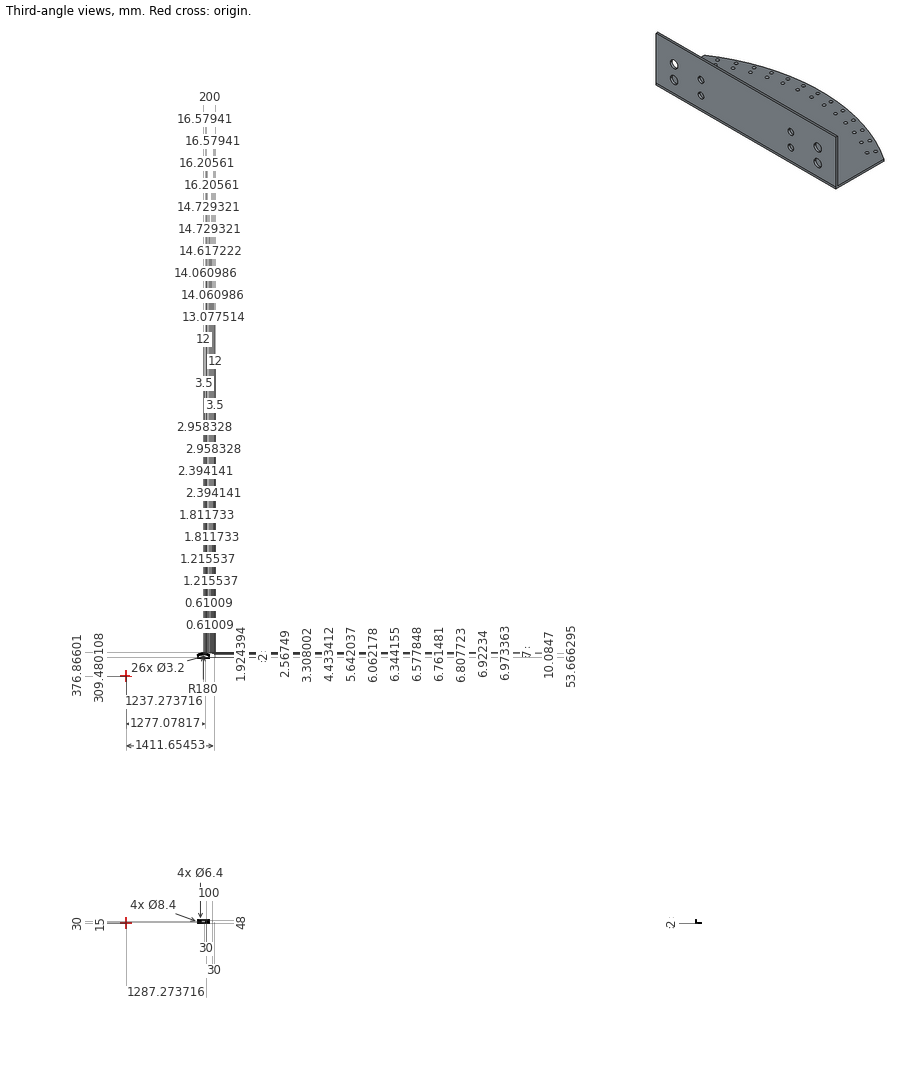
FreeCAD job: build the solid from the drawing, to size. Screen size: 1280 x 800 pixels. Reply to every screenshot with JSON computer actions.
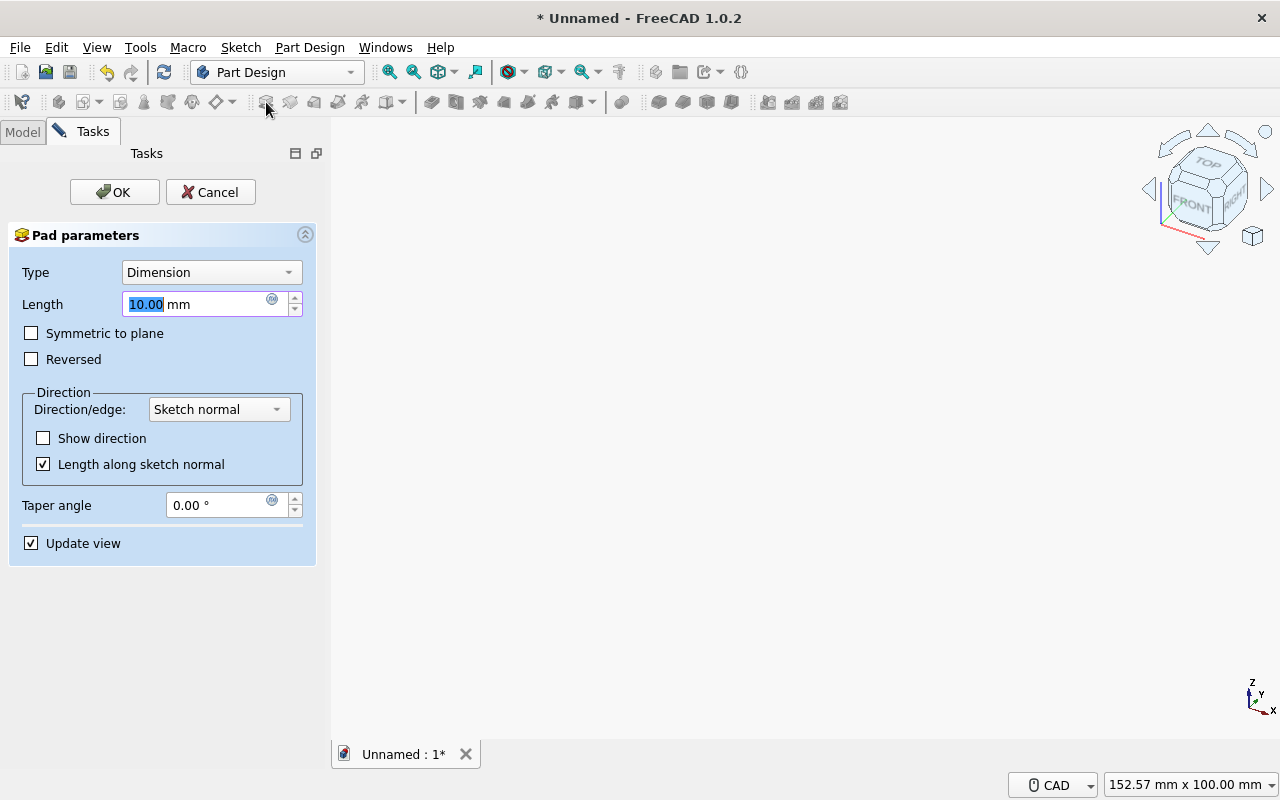
{"action": "type", "text": "2"}
{"action": "key", "text": "Tab"}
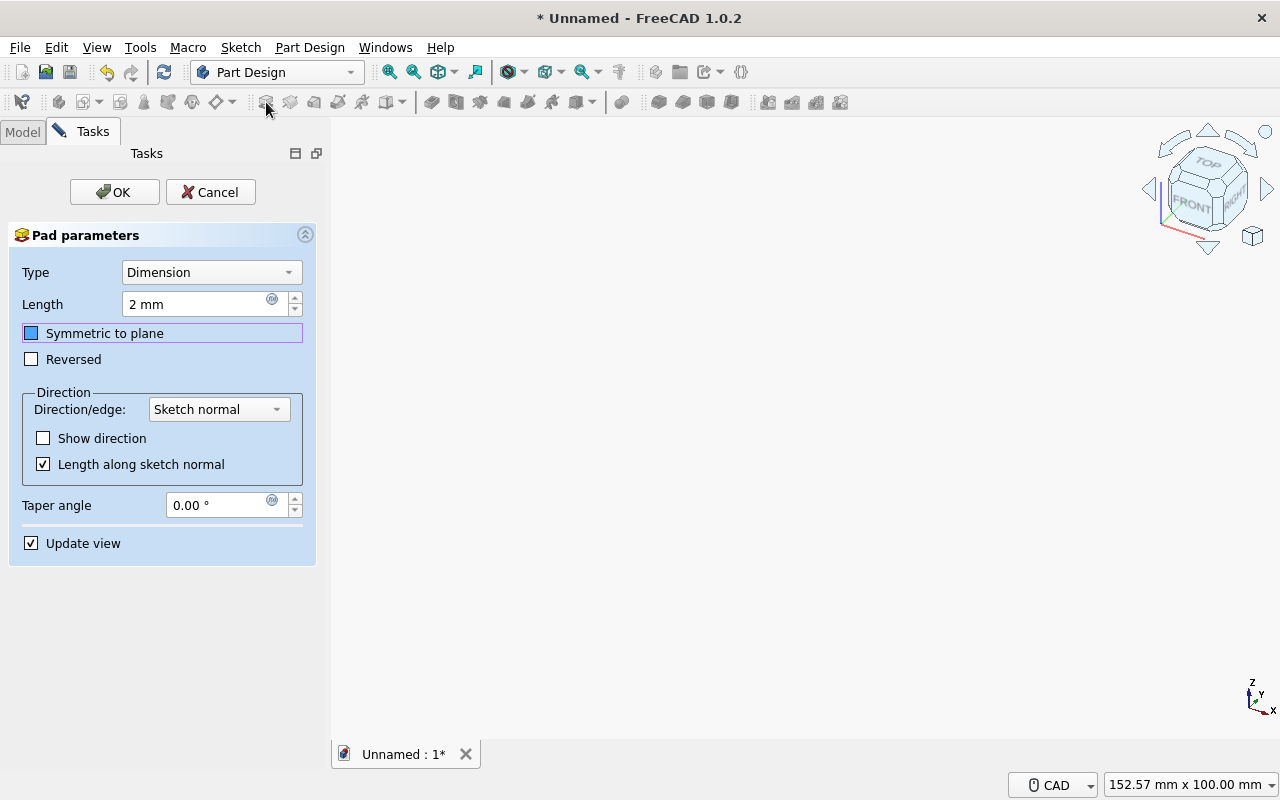
{"action": "left_click", "coordinate": [115, 192]}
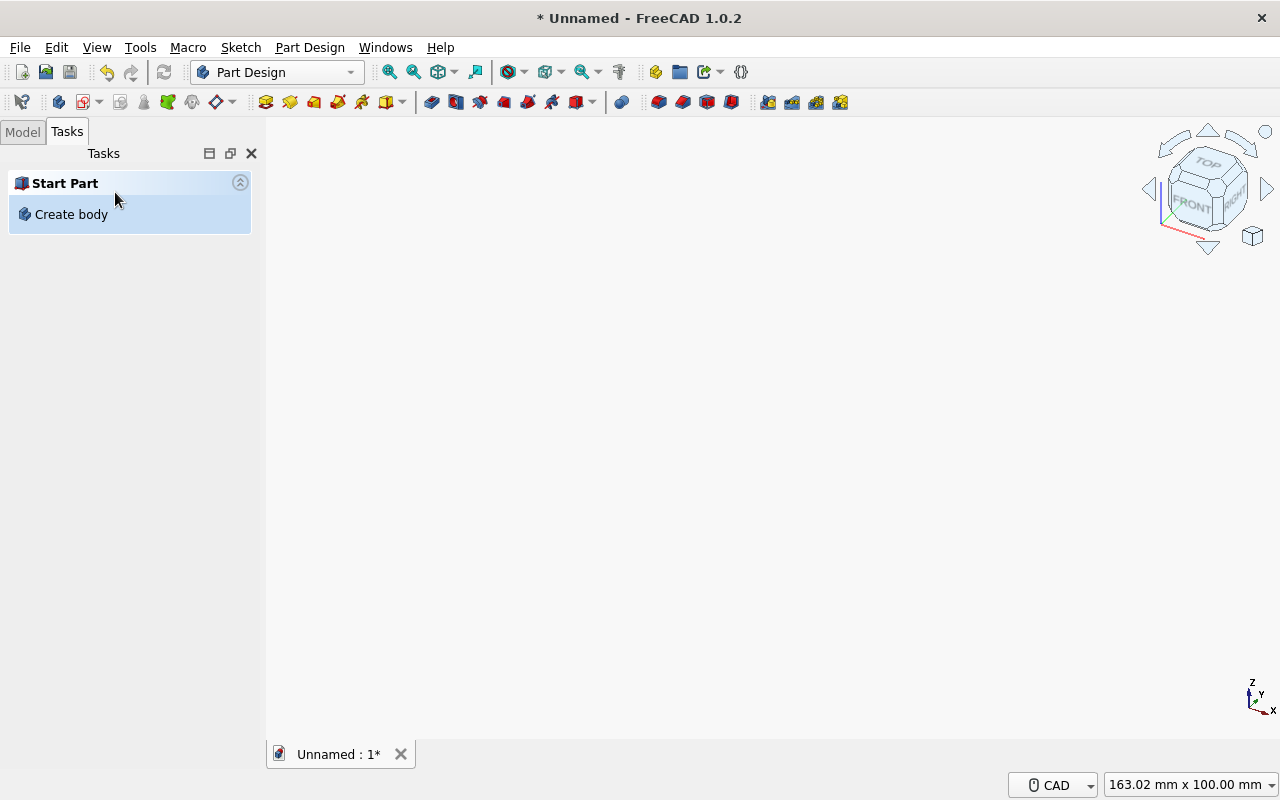
{"action": "key", "text": "v f"}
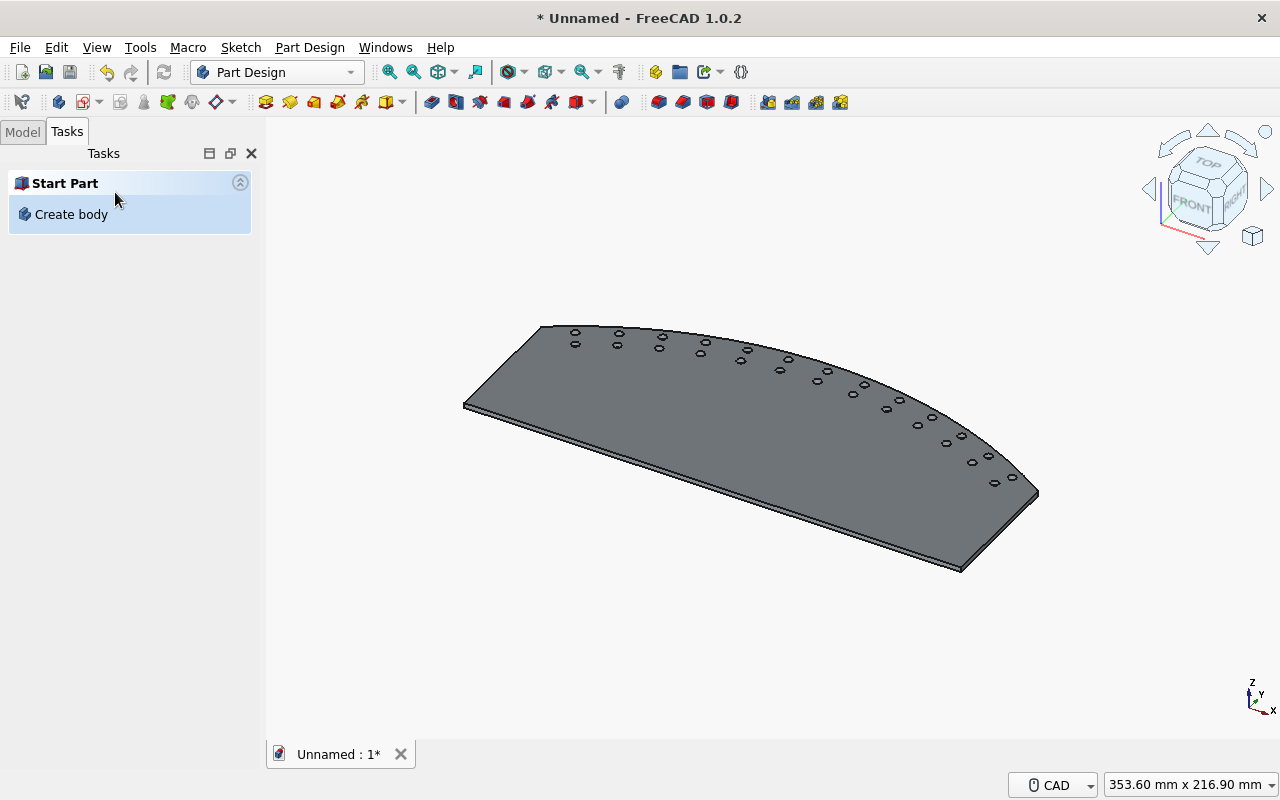
{"action": "left_click", "coordinate": [827, 465]}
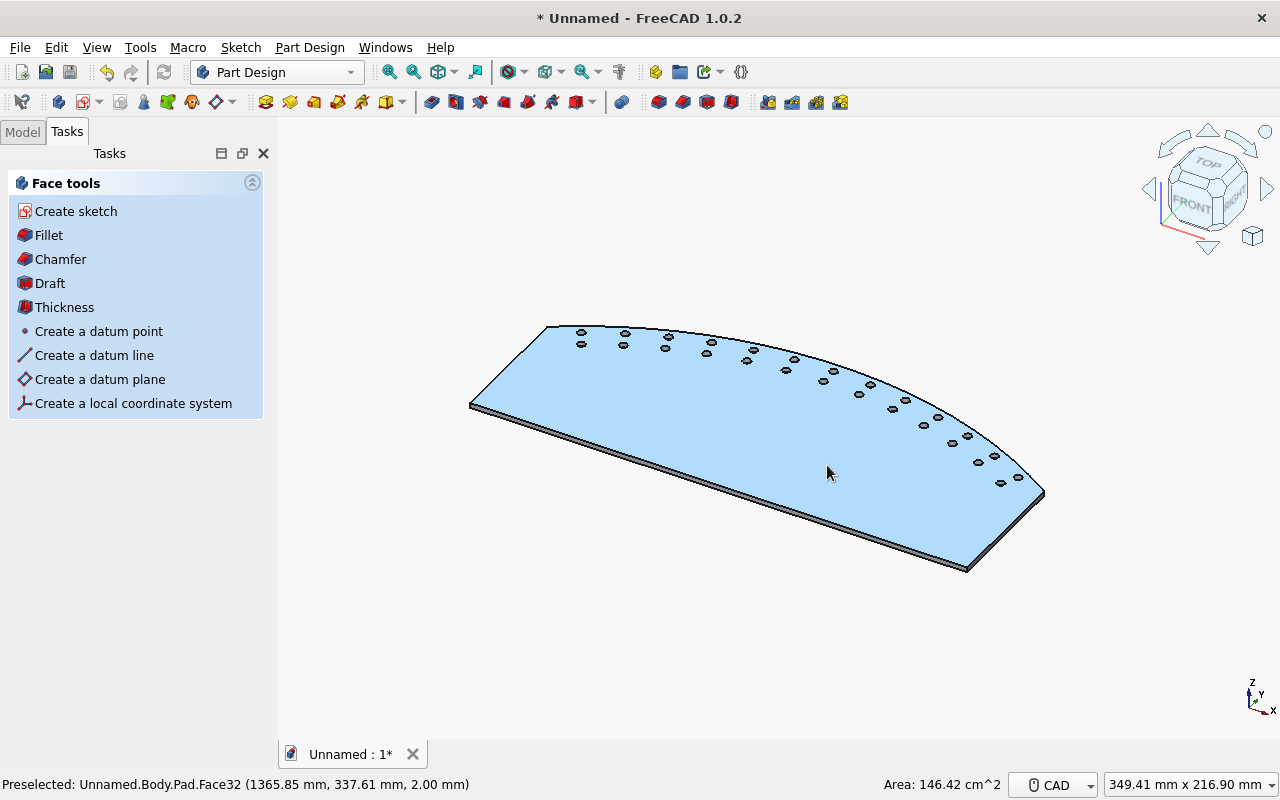
{"action": "left_click", "coordinate": [84, 102]}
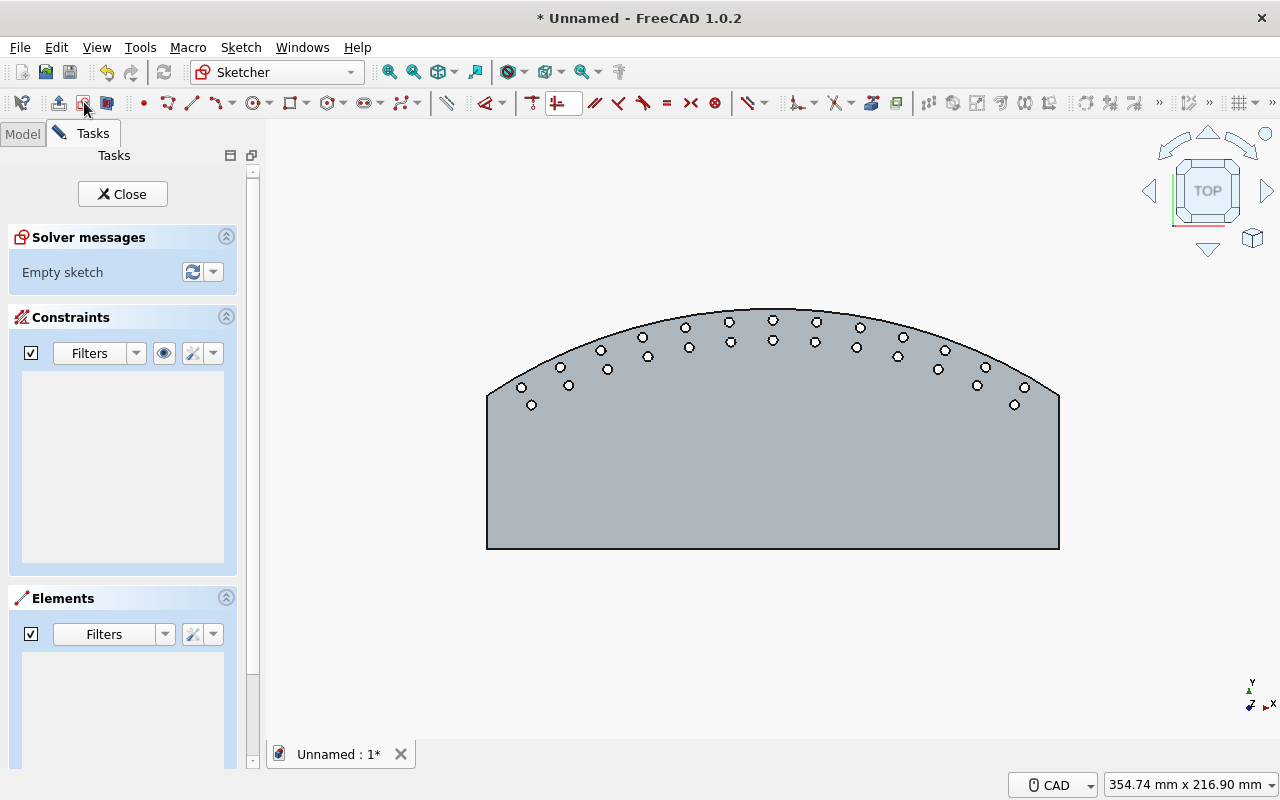
{"action": "left_click", "coordinate": [290, 104]}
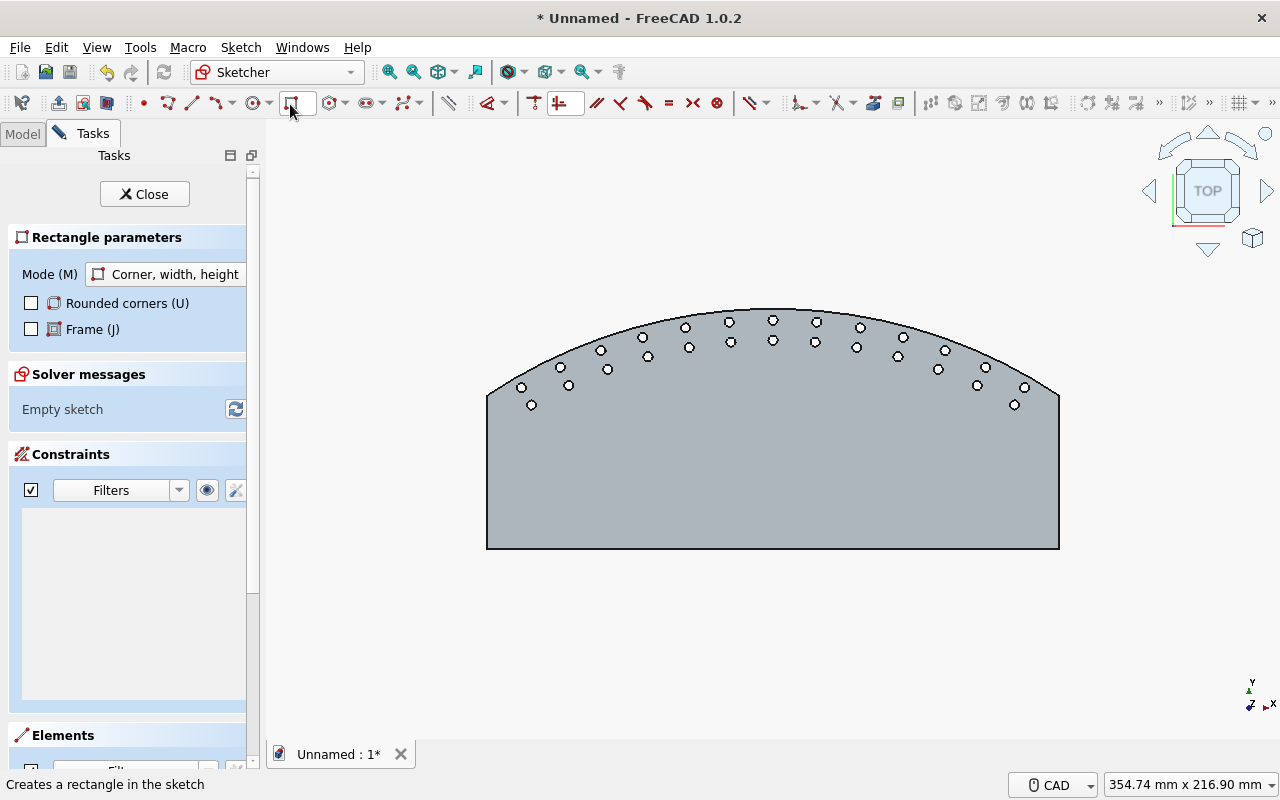
{"action": "scroll", "coordinate": [487, 543], "scroll_direction": "up", "scroll_amount": 6}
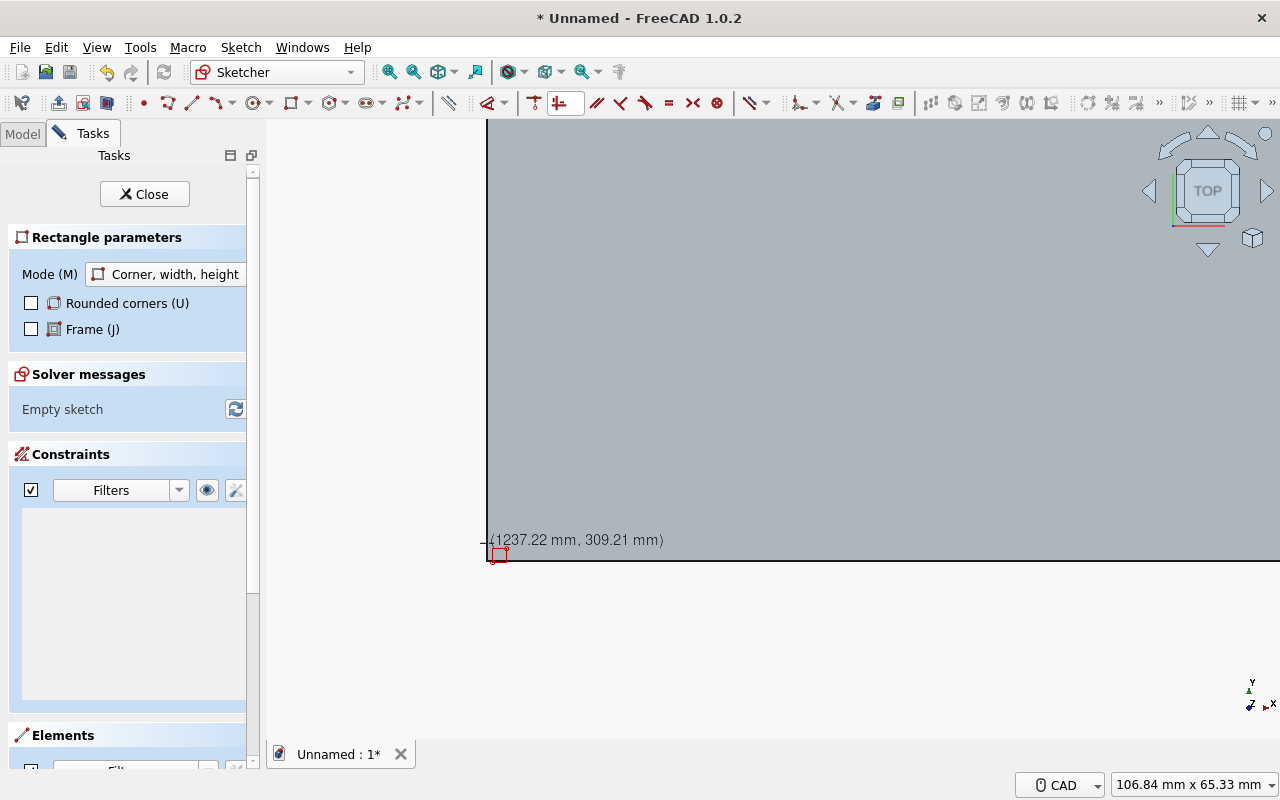
{"action": "left_click", "coordinate": [487, 542]}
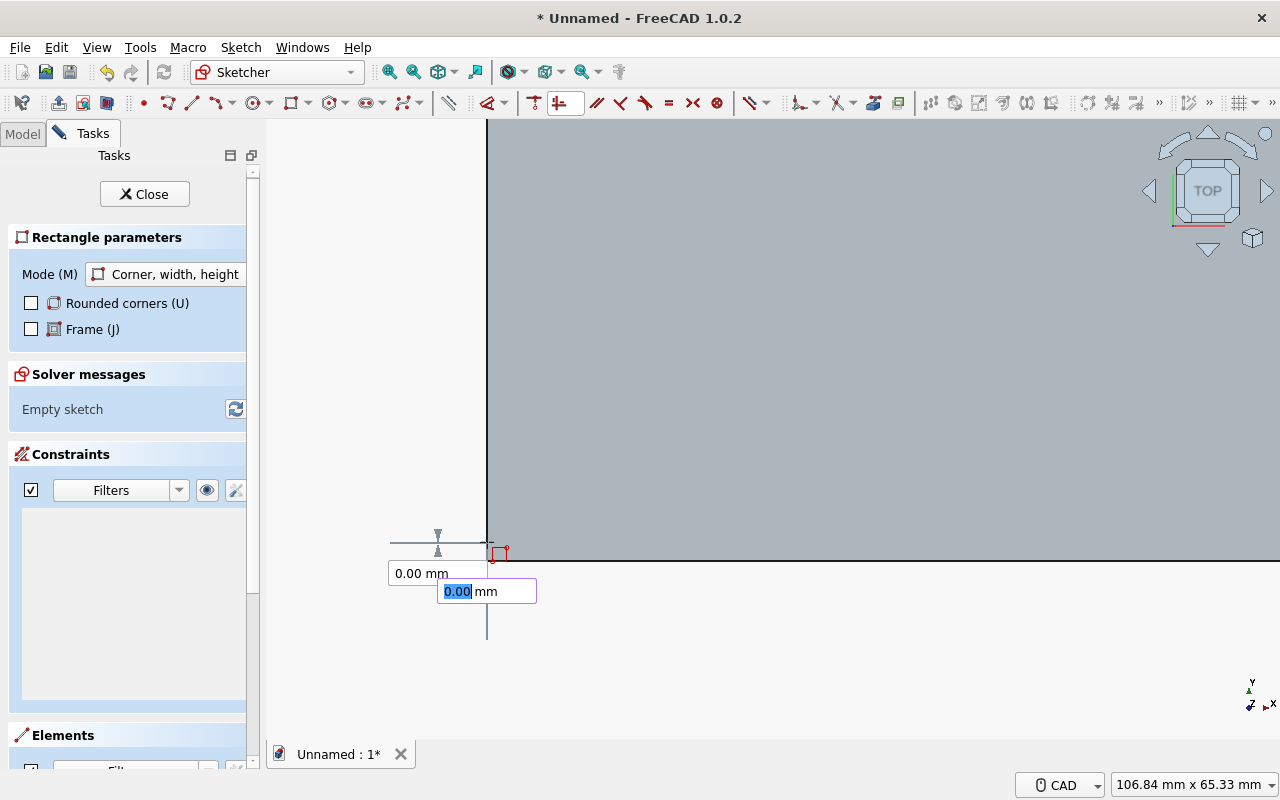
{"action": "scroll", "coordinate": [389, 376], "scroll_direction": "down", "scroll_amount": 6}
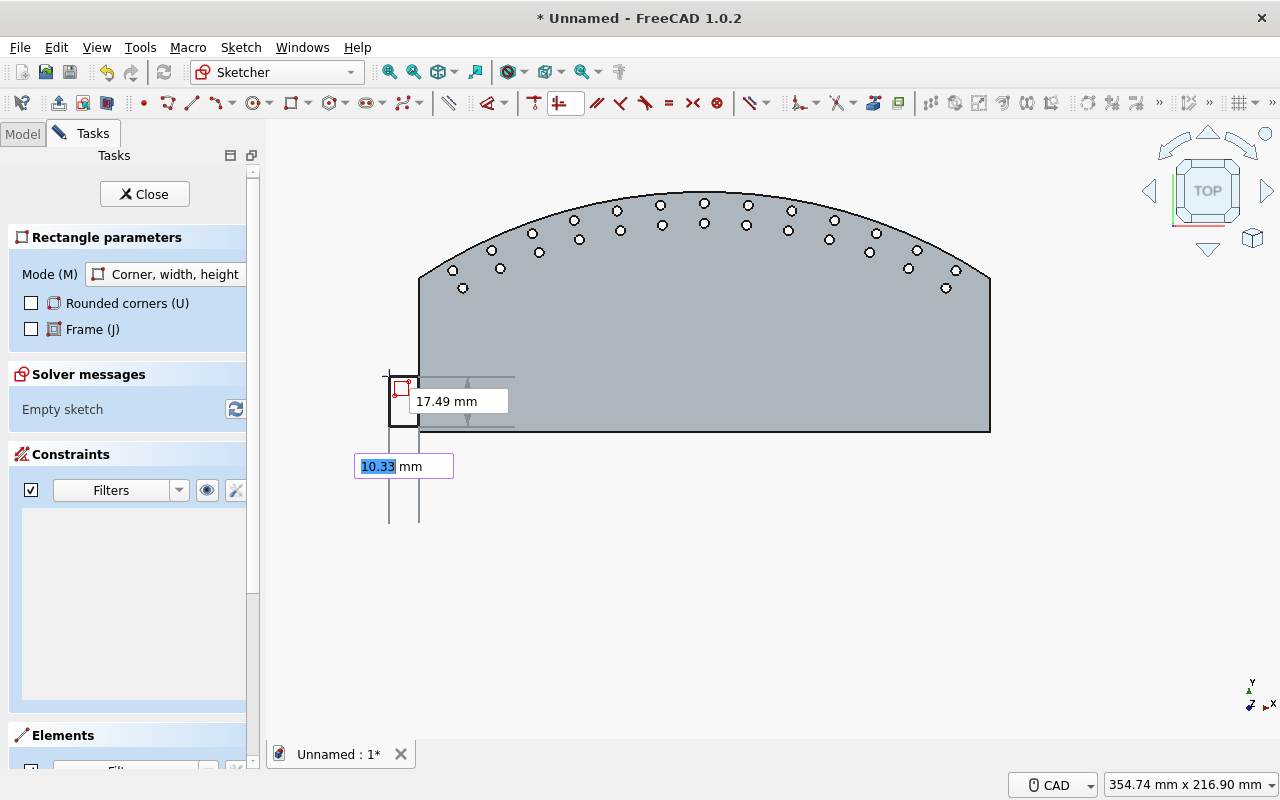
{"action": "left_click", "coordinate": [990, 432]}
{"action": "key", "text": "Escape"}